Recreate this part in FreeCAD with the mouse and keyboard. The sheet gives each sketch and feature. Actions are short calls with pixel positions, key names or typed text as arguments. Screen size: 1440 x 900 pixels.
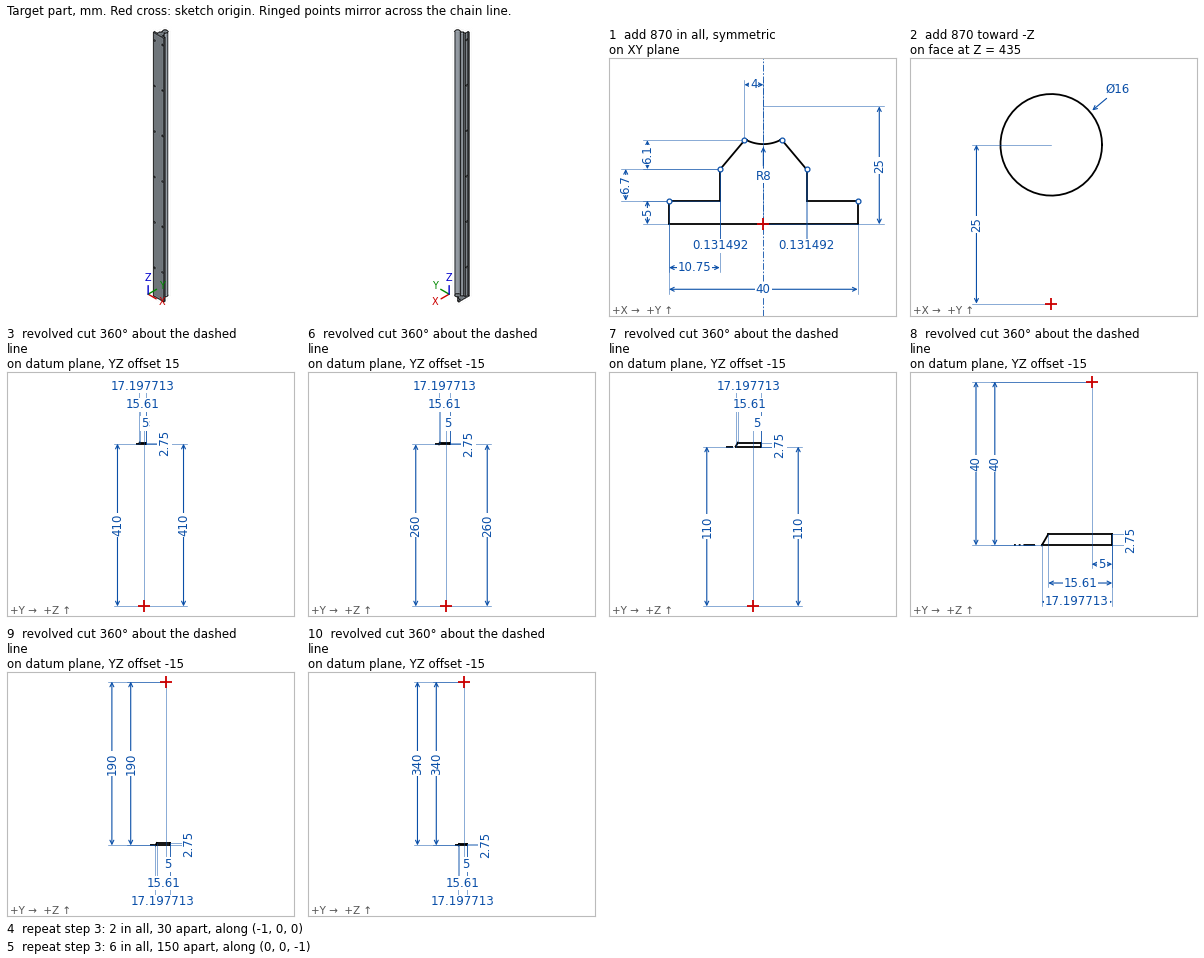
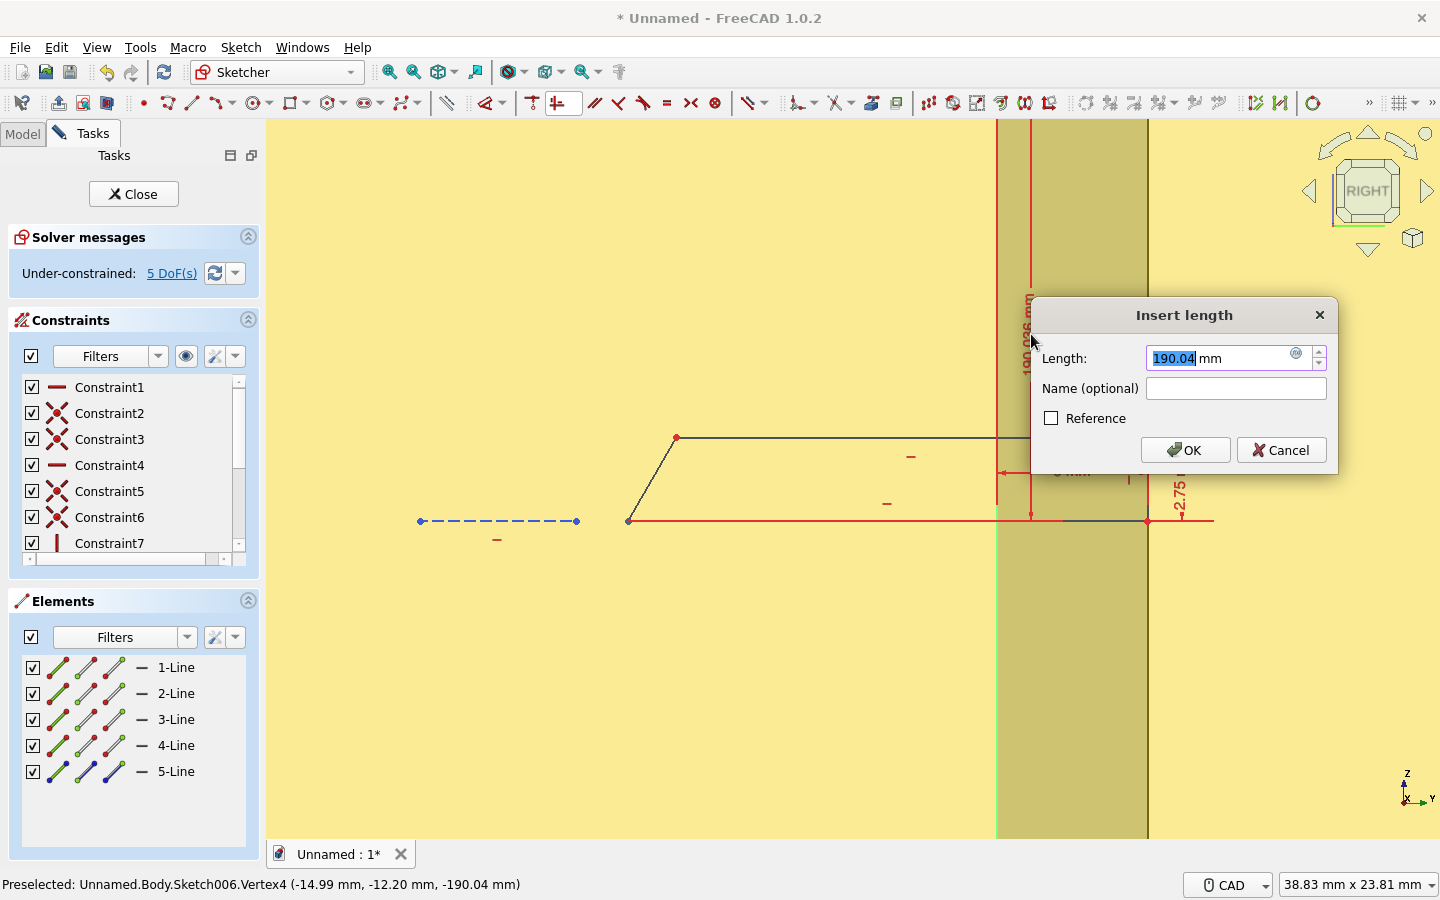
text(190)
key(Return)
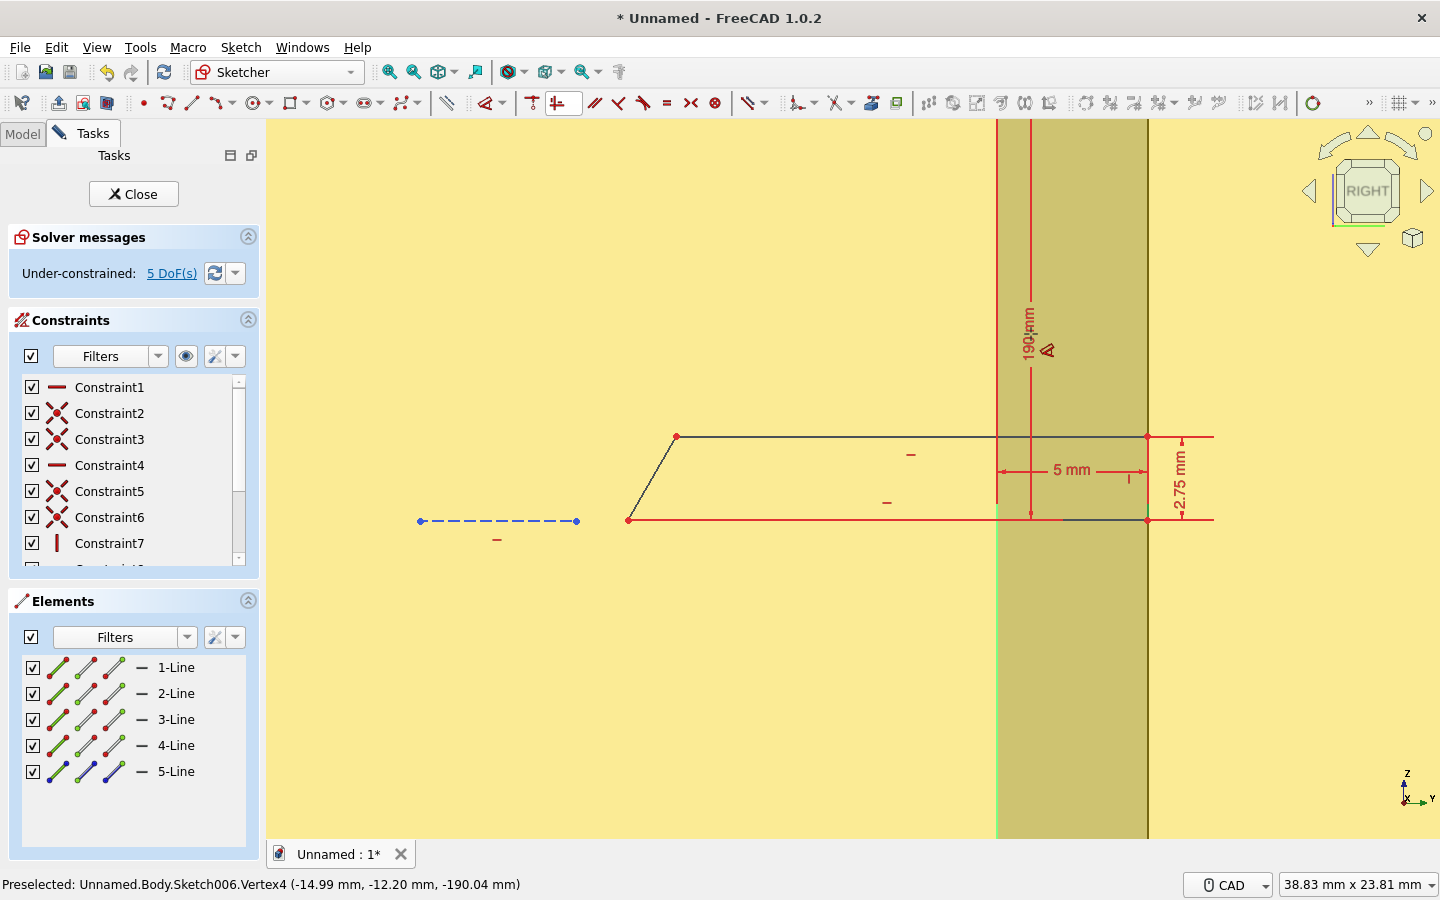
click(576, 521)
click(1031, 248)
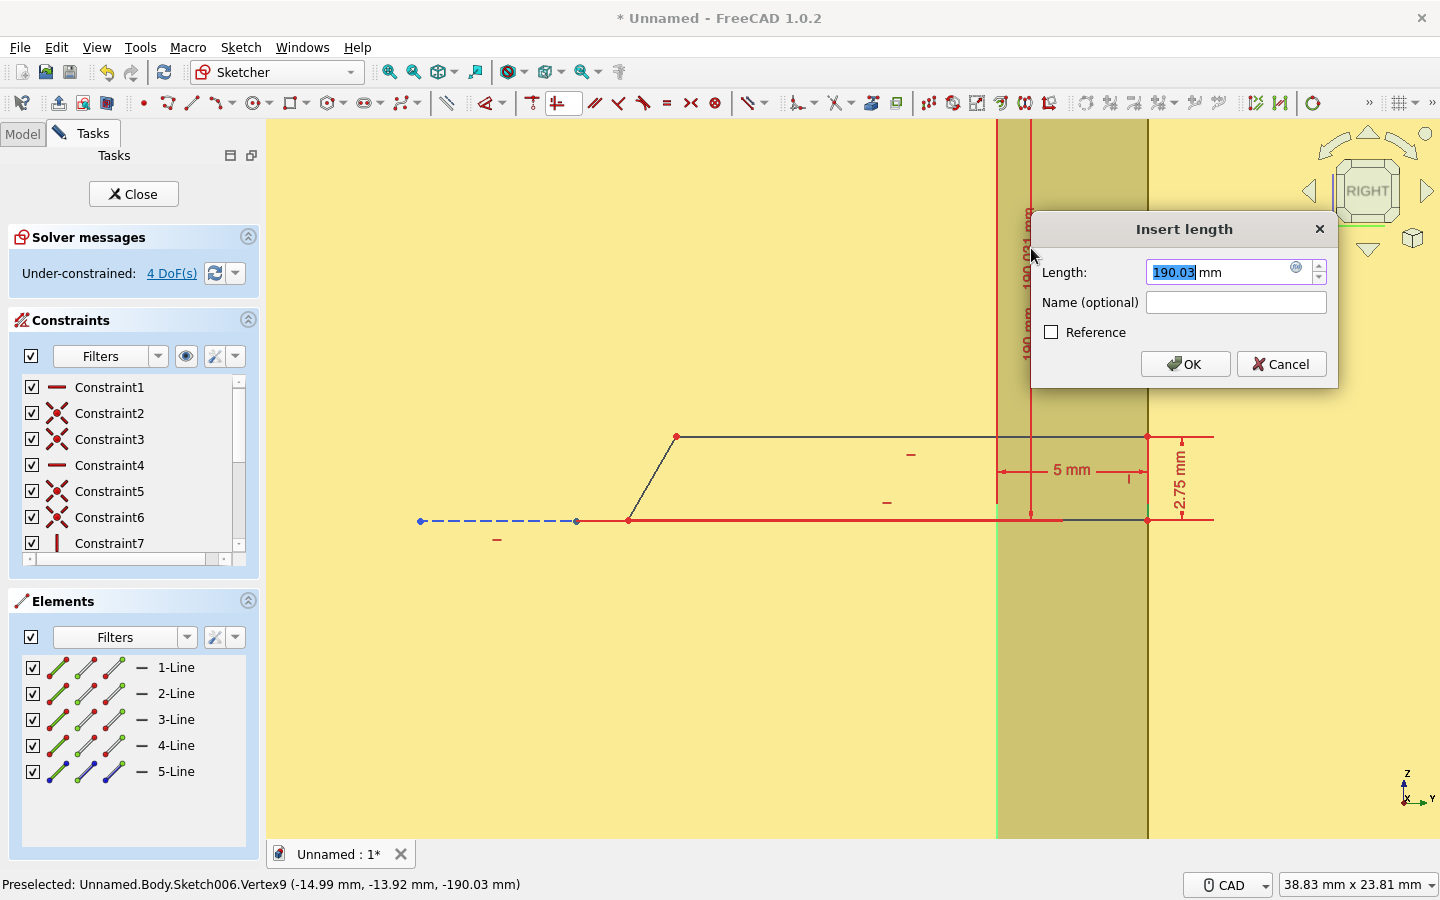
text(190)
key(Return)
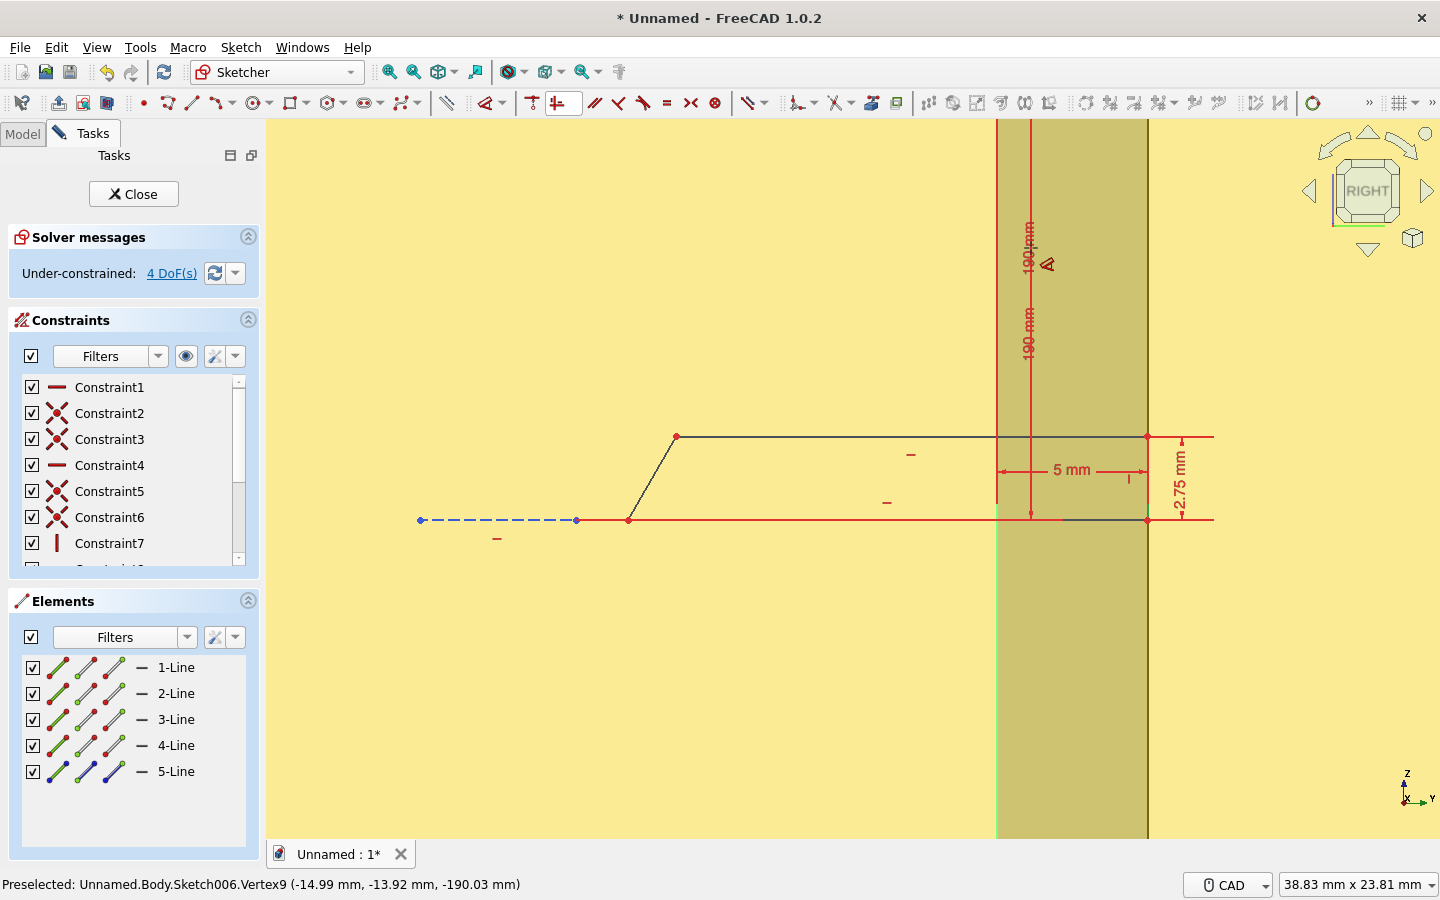
scroll(1006, 437, up, 2)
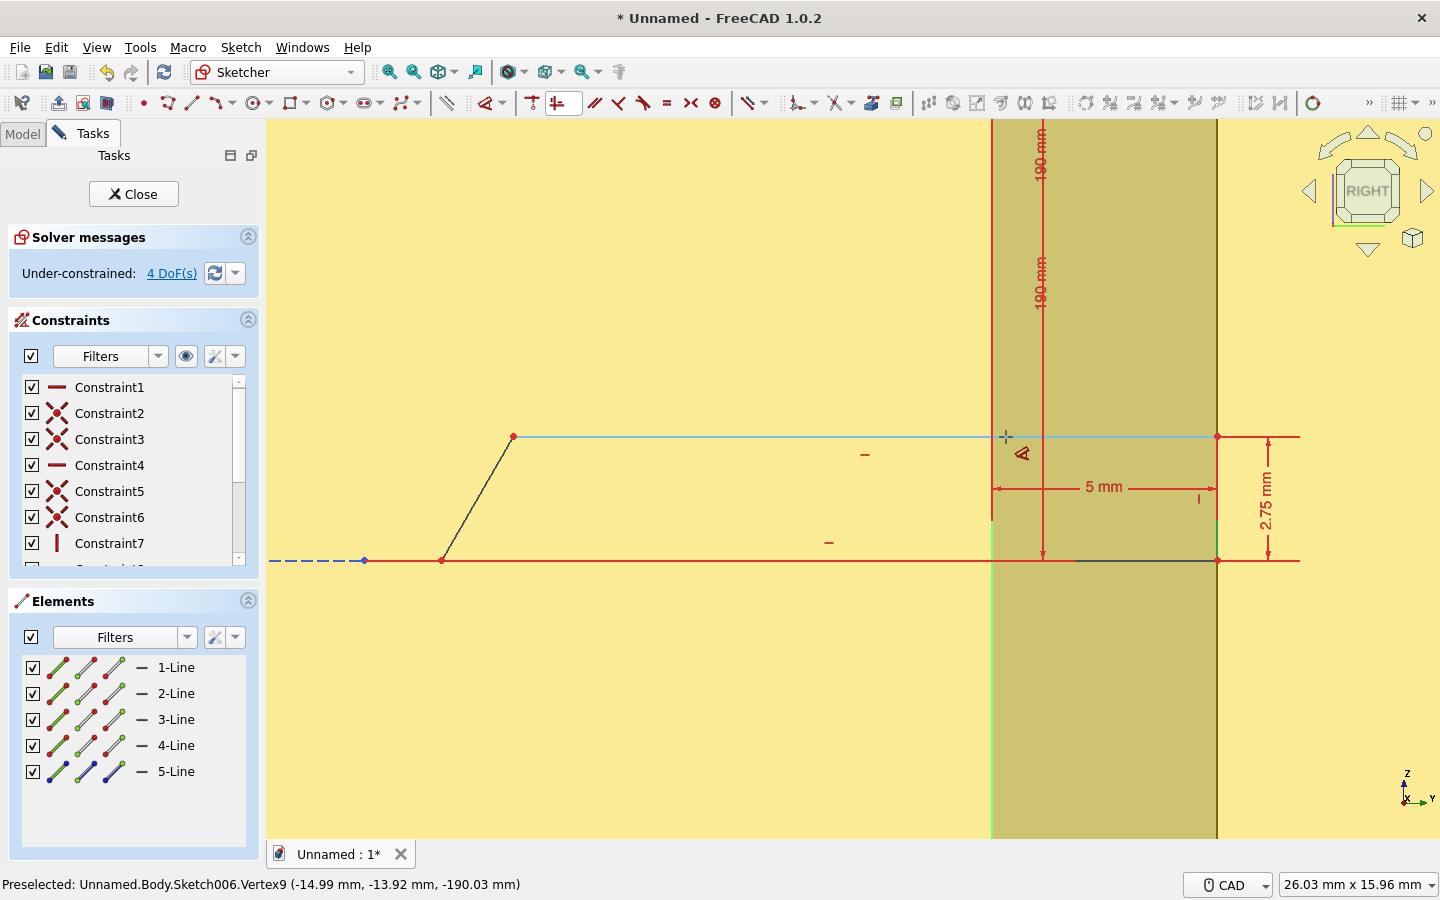
click(1006, 437)
click(865, 403)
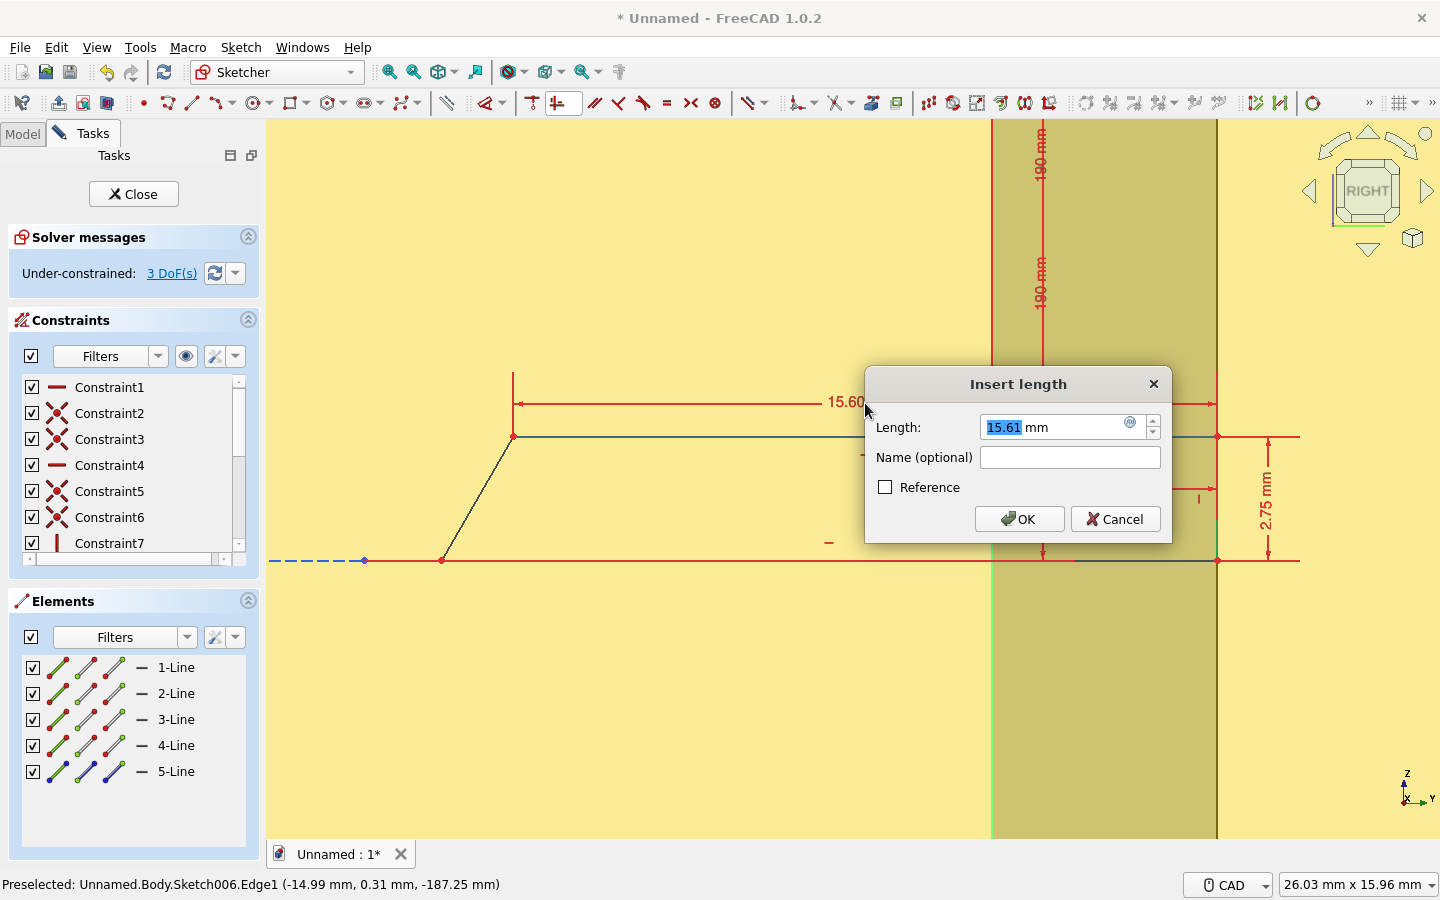
text(15.61)
key(Return)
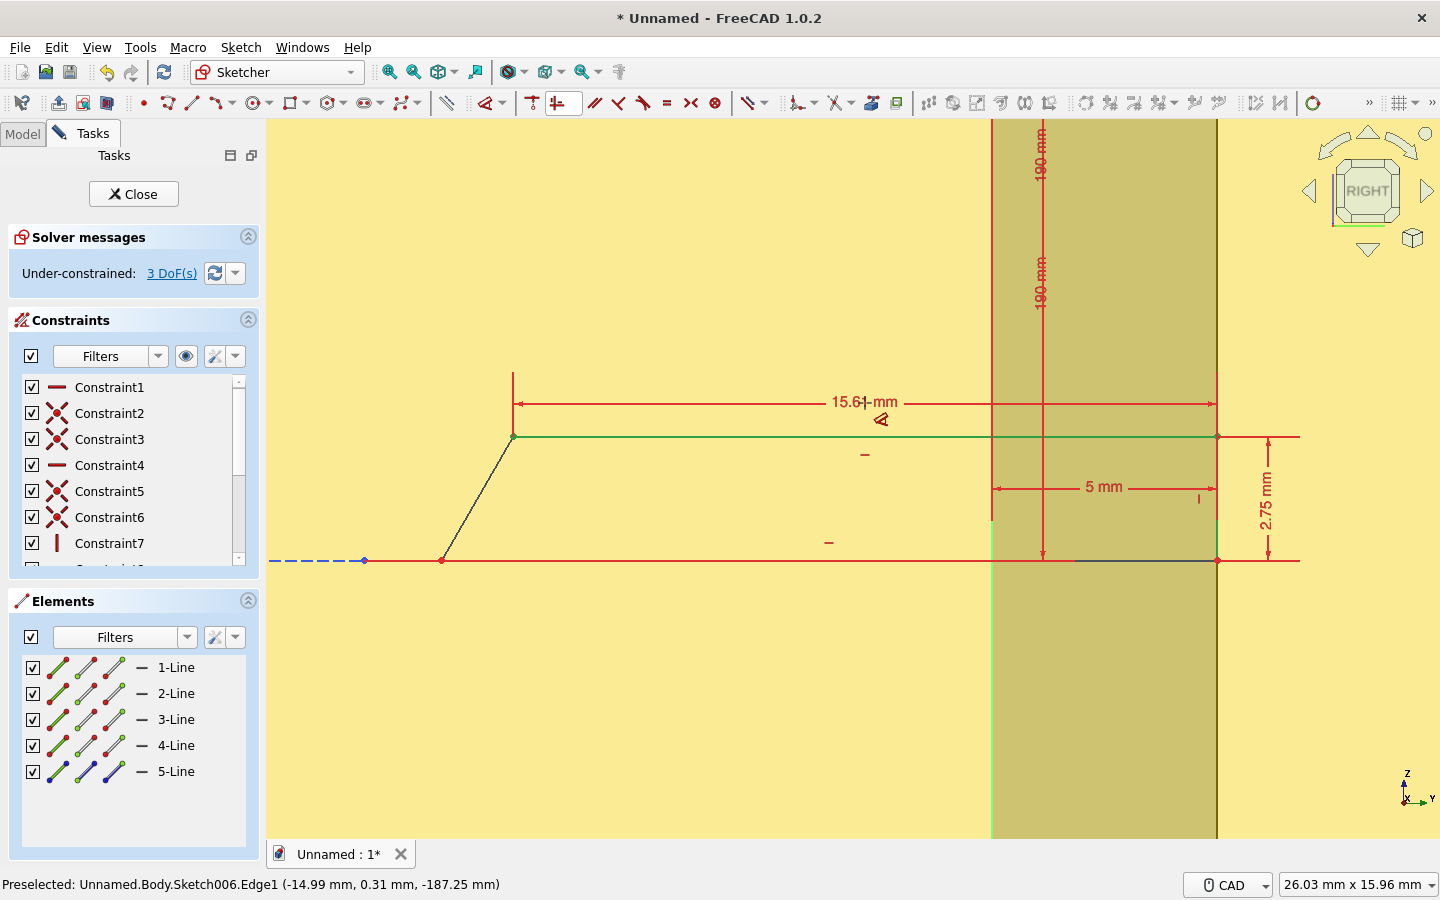
click(674, 561)
click(830, 595)